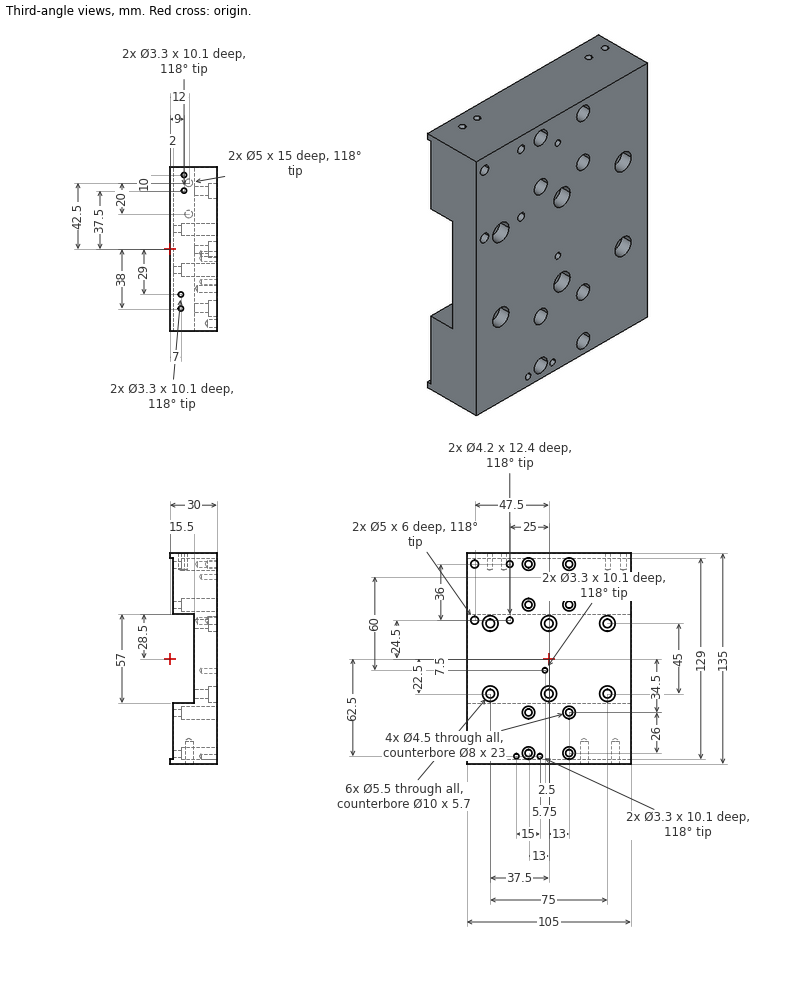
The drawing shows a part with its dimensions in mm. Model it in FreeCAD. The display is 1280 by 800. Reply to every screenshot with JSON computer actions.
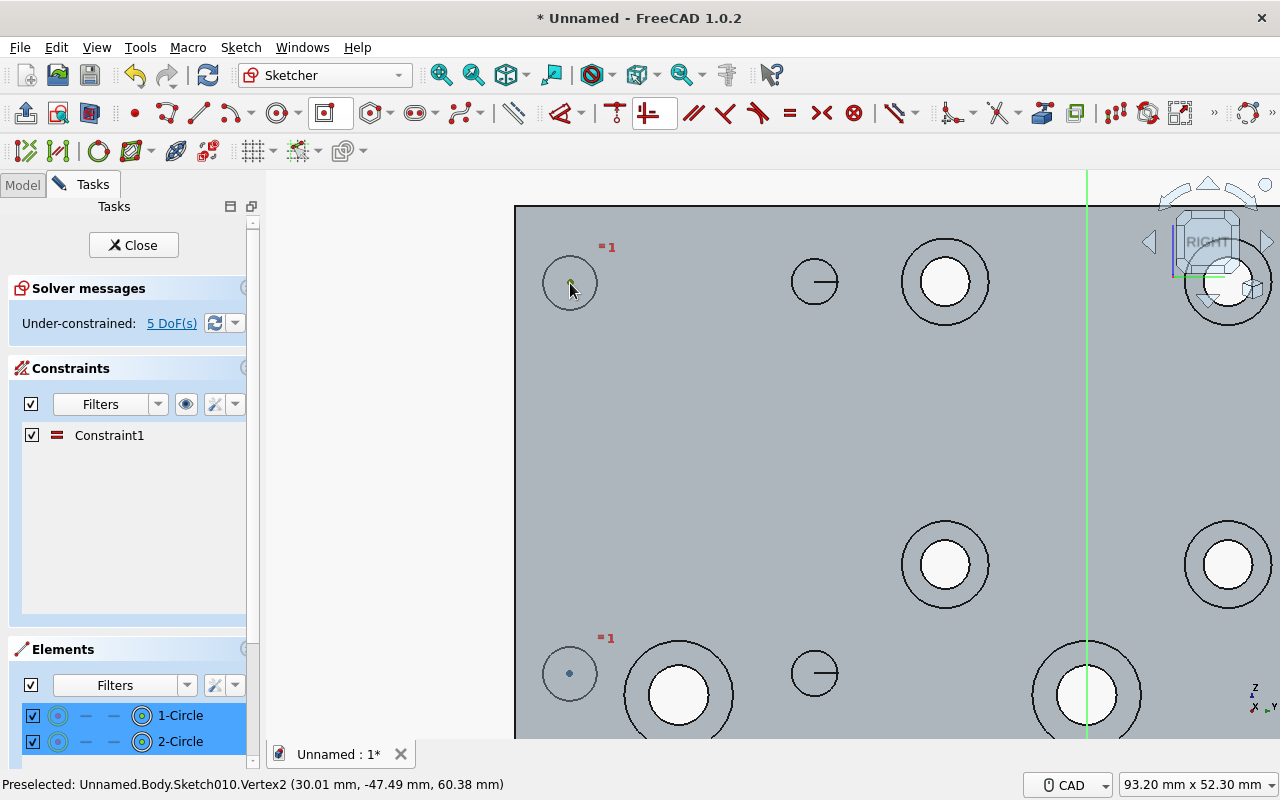
{"action": "left_click", "coordinate": [672, 114]}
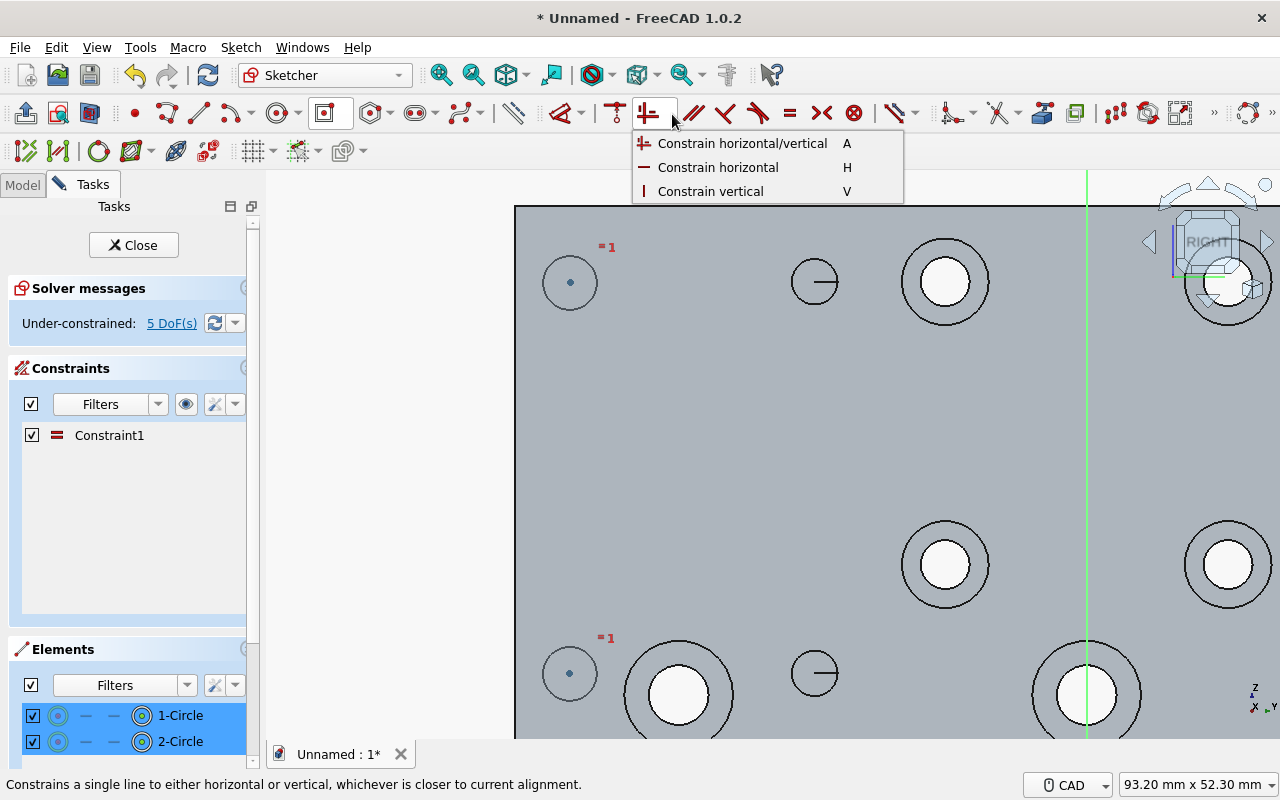
{"action": "left_click", "coordinate": [768, 191]}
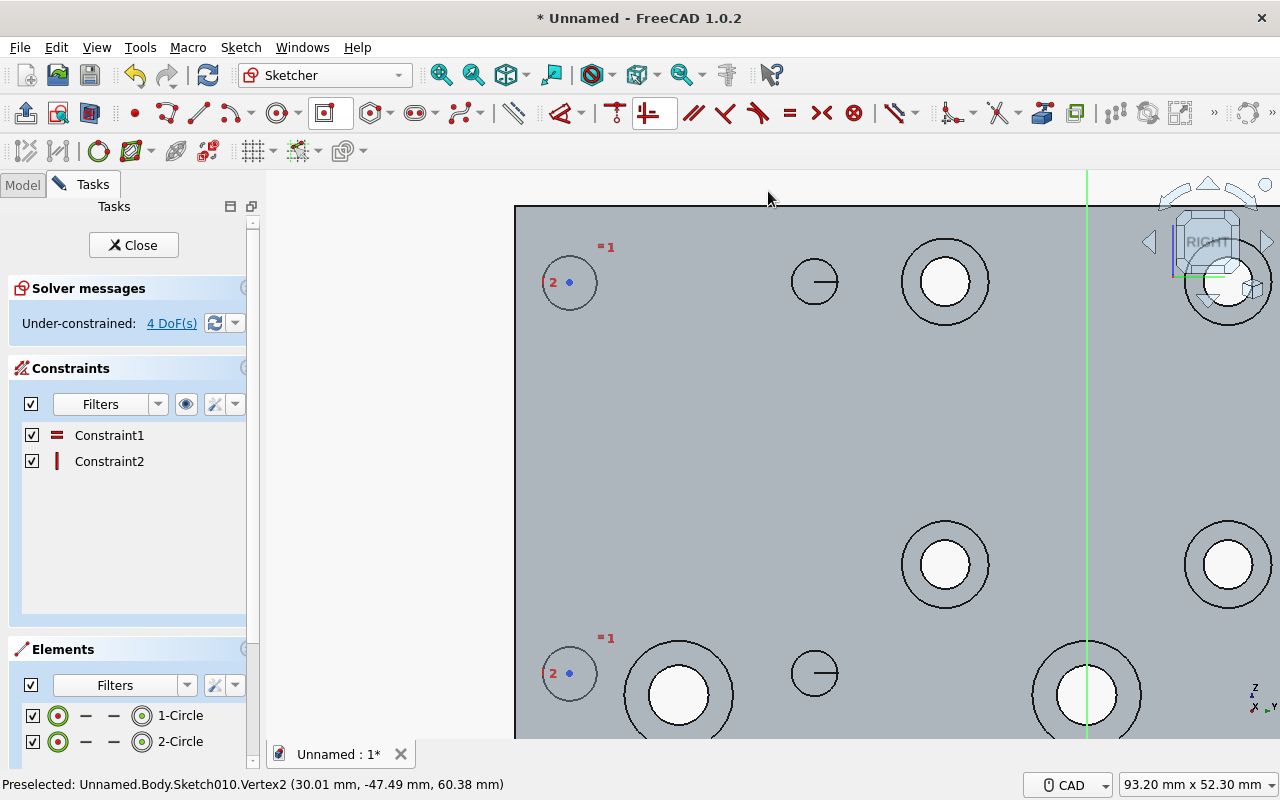
{"action": "left_click", "coordinate": [560, 114]}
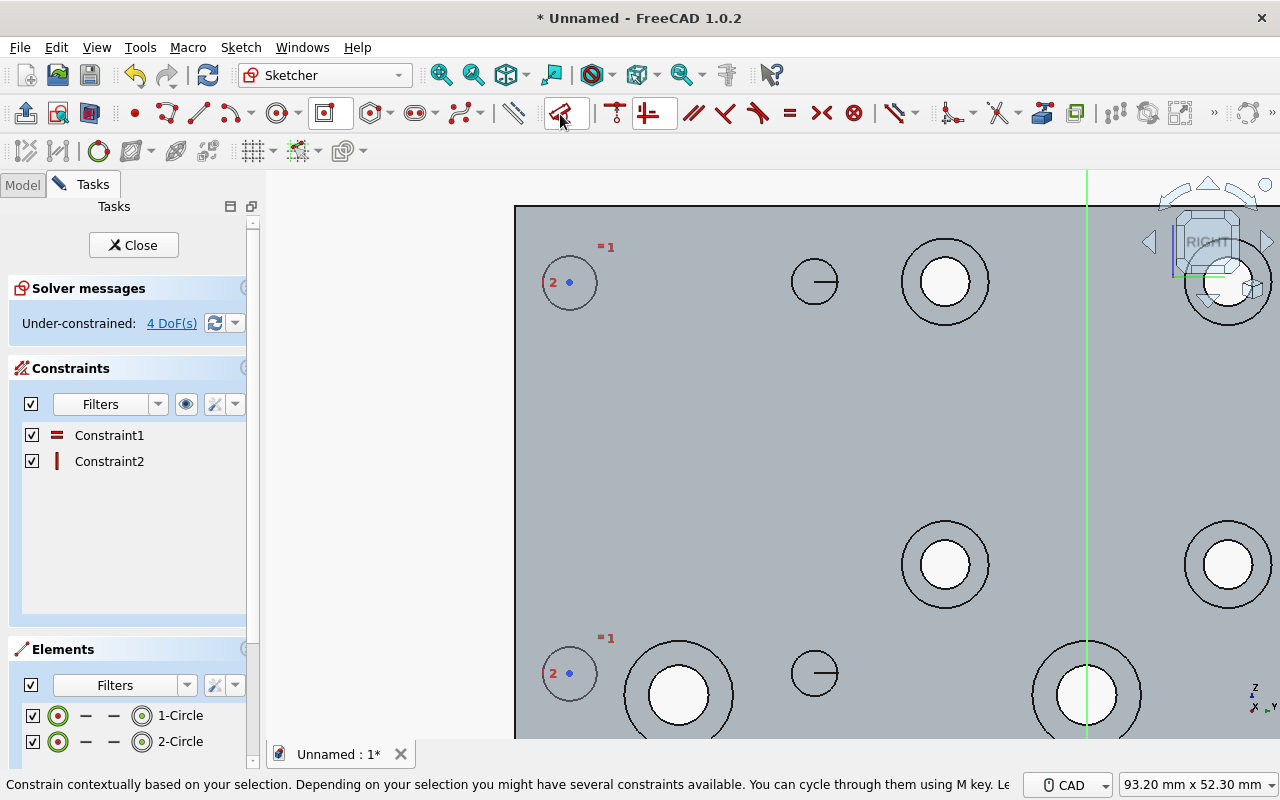
{"action": "left_click", "coordinate": [589, 655]}
{"action": "left_click", "coordinate": [612, 633]}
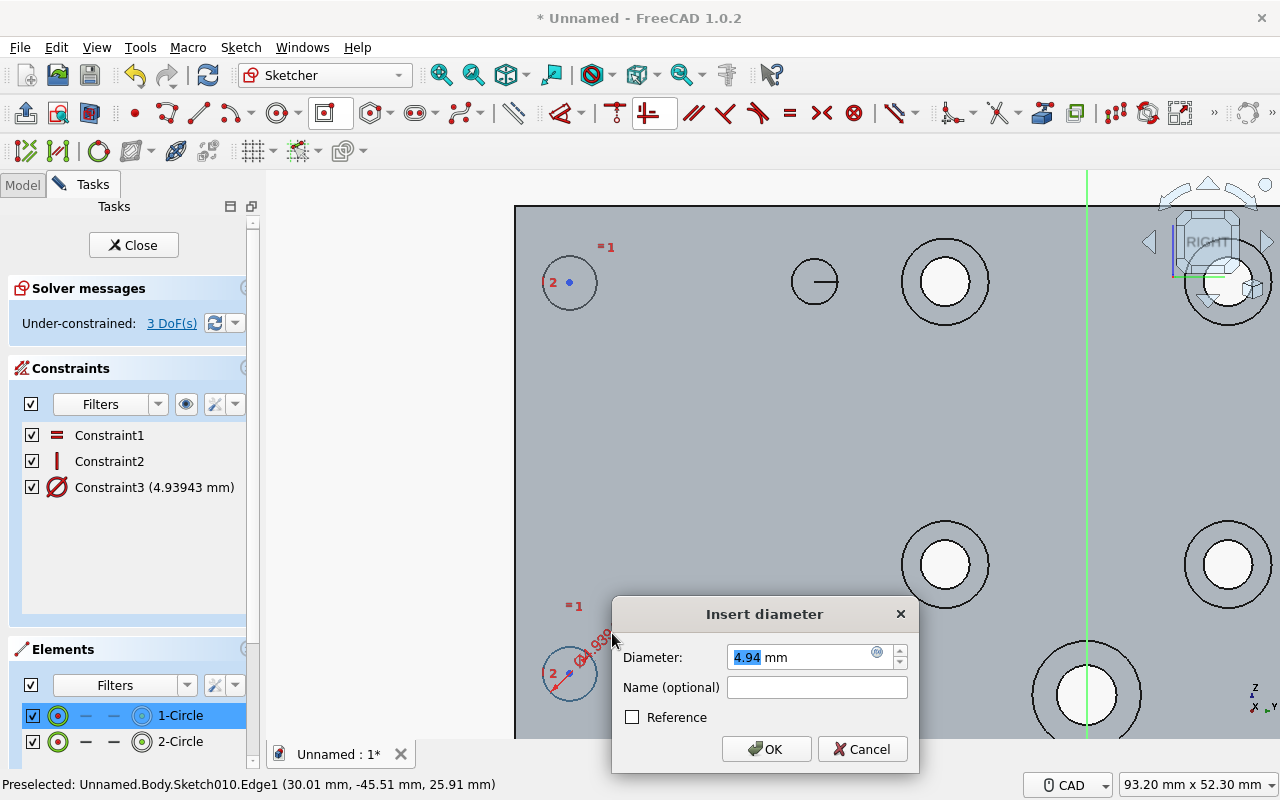
{"action": "type", "text": "5"}
{"action": "key", "text": "Return"}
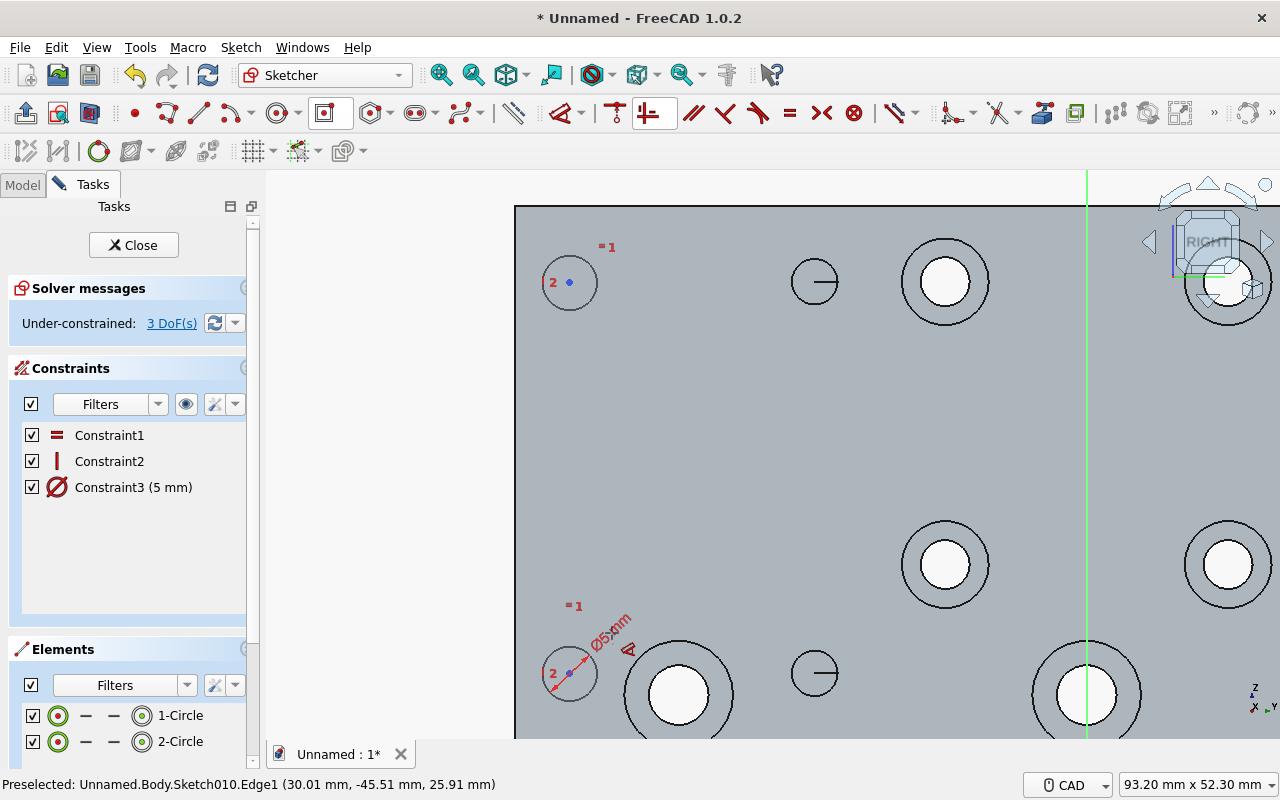
{"action": "left_click", "coordinate": [570, 674]}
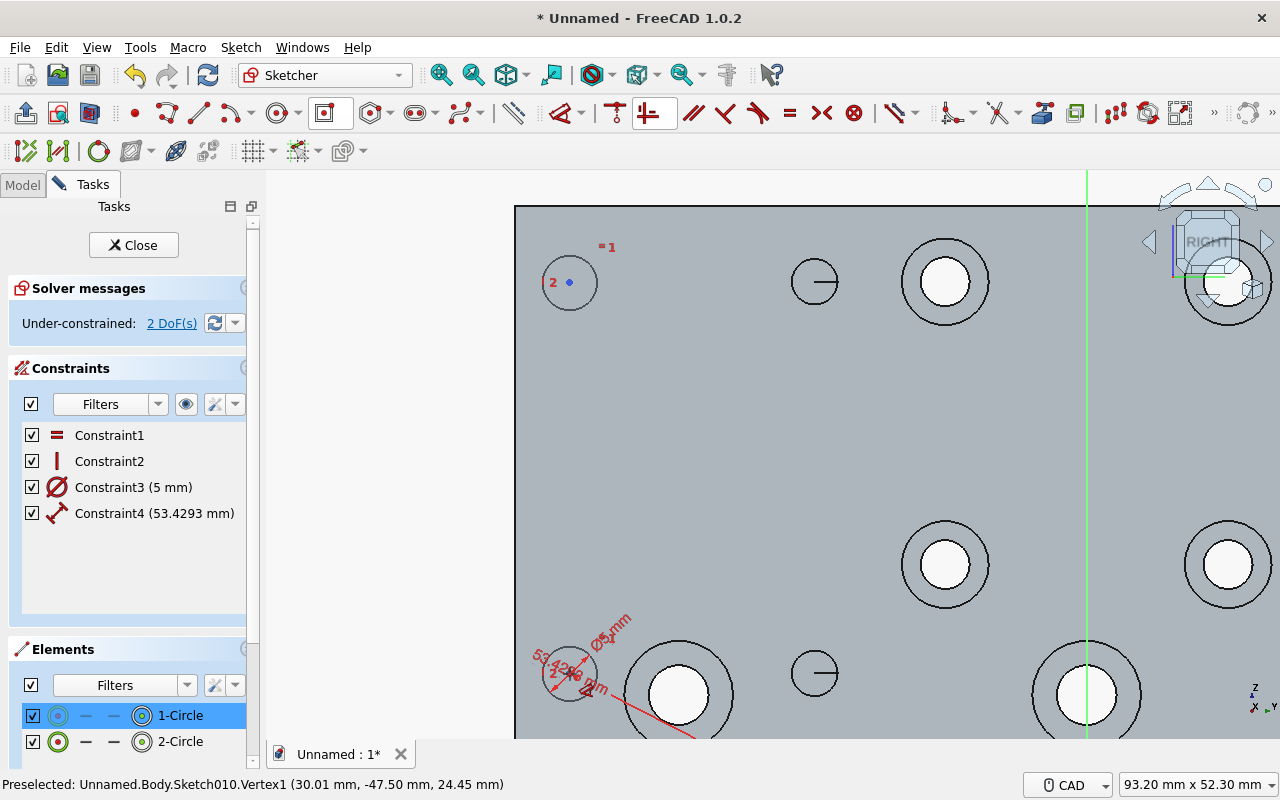
{"action": "left_click", "coordinate": [570, 283]}
{"action": "left_click", "coordinate": [536, 478]}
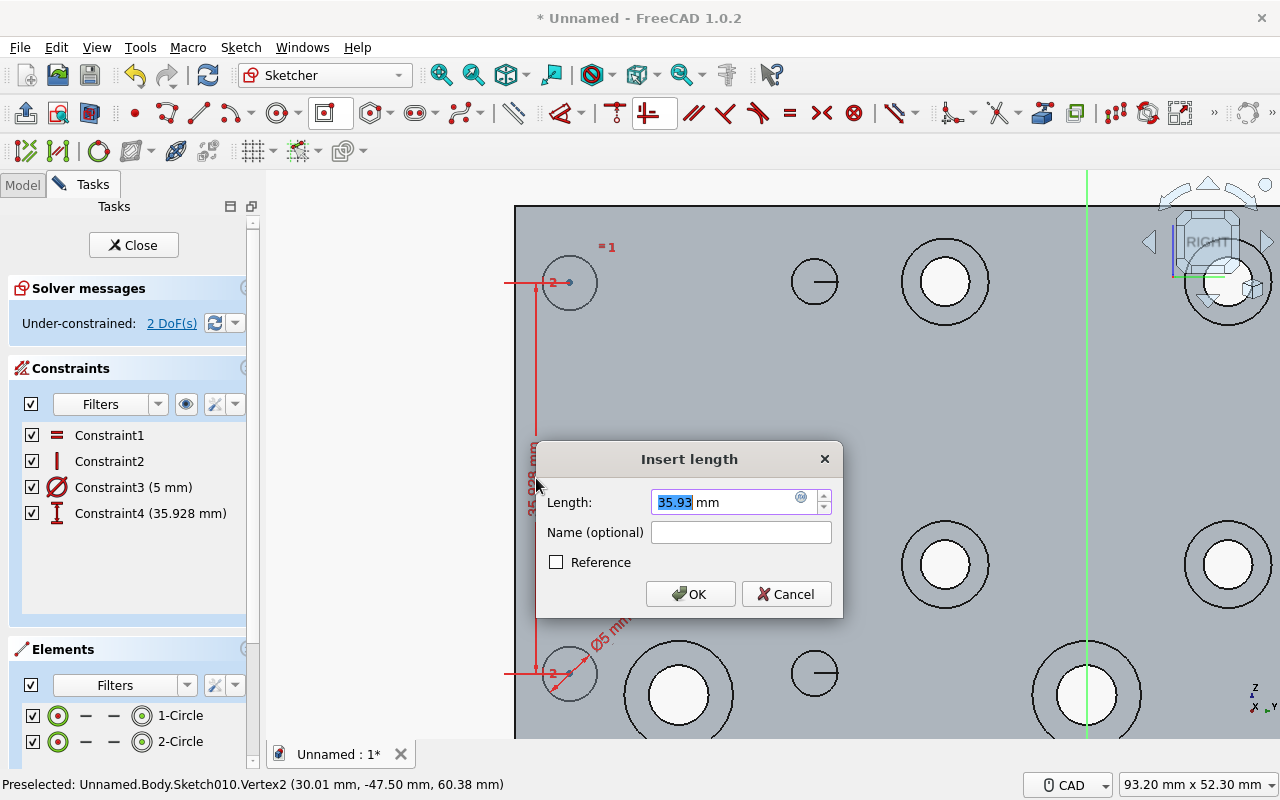
{"action": "type", "text": "36"}
{"action": "key", "text": "Return"}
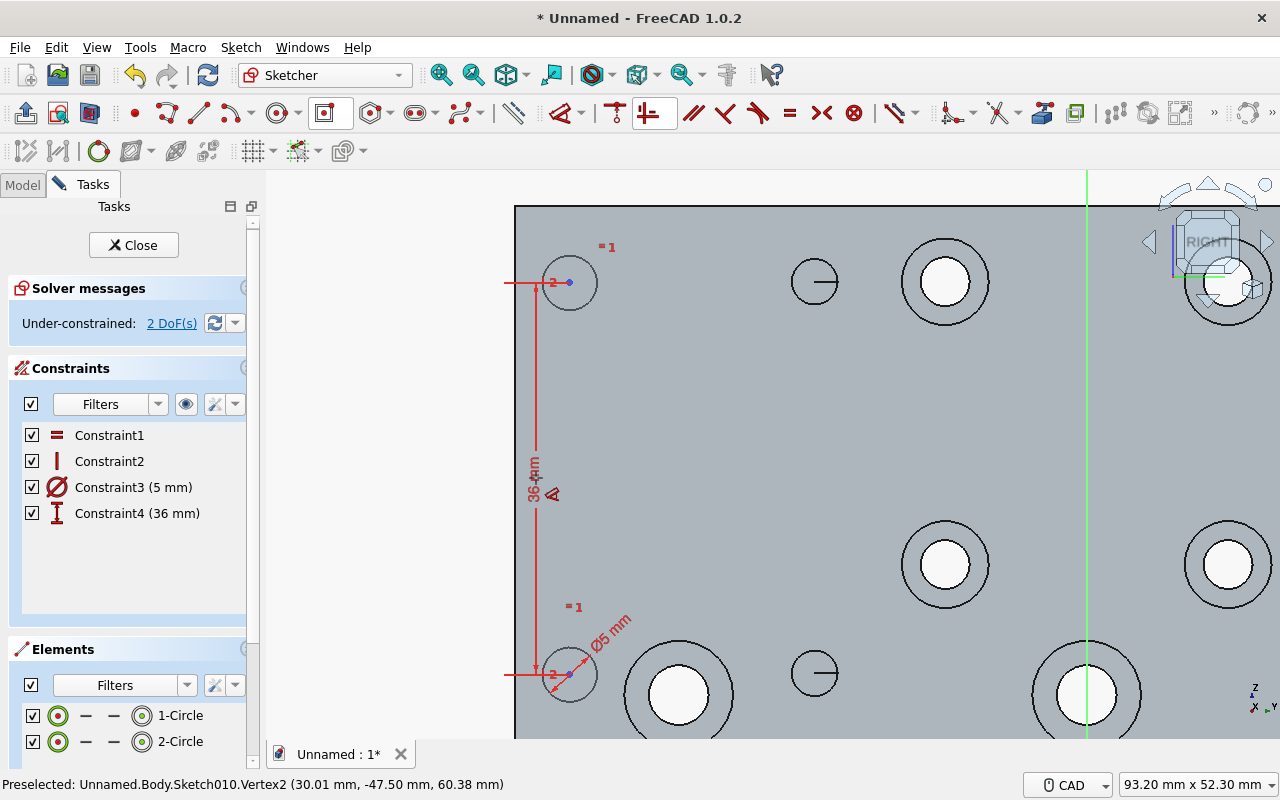
{"action": "left_click", "coordinate": [570, 675]}
{"action": "left_click", "coordinate": [828, 641]}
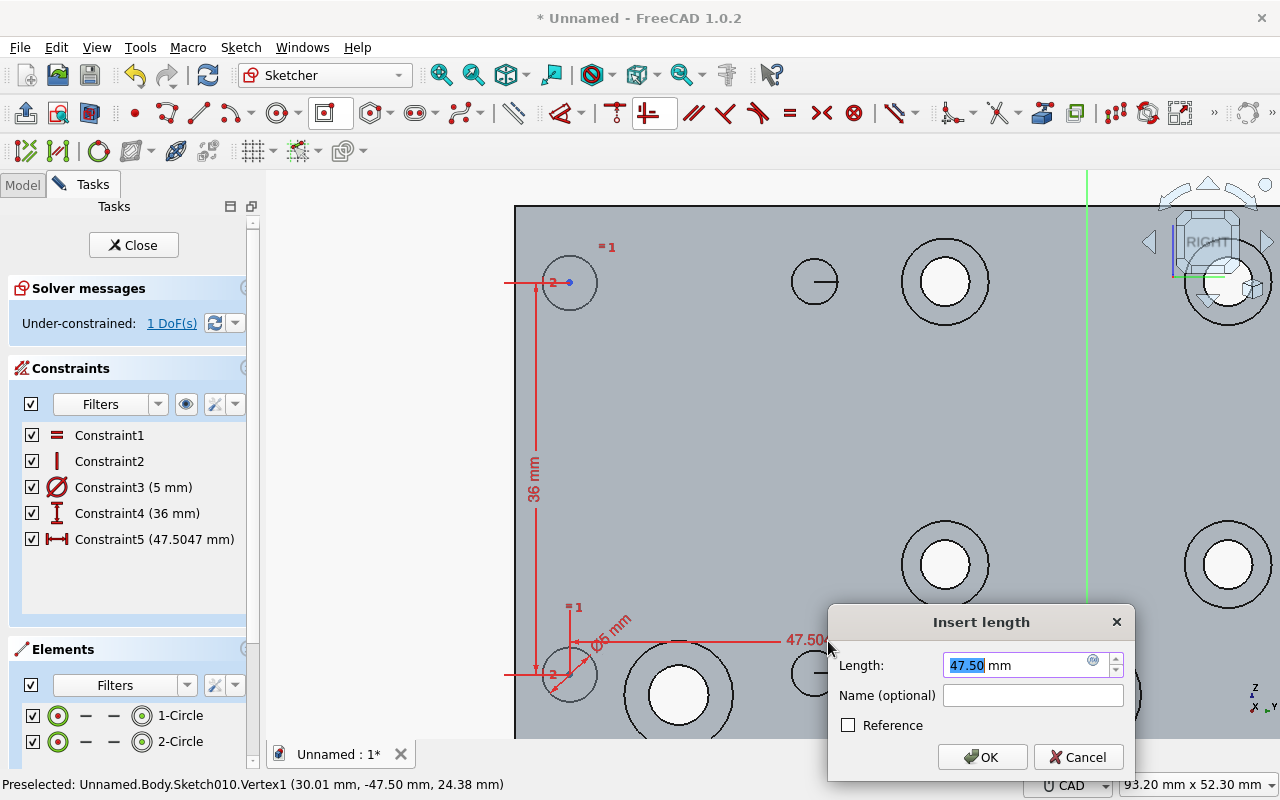
{"action": "type", "text": "47.5"}
{"action": "key", "text": "Return"}